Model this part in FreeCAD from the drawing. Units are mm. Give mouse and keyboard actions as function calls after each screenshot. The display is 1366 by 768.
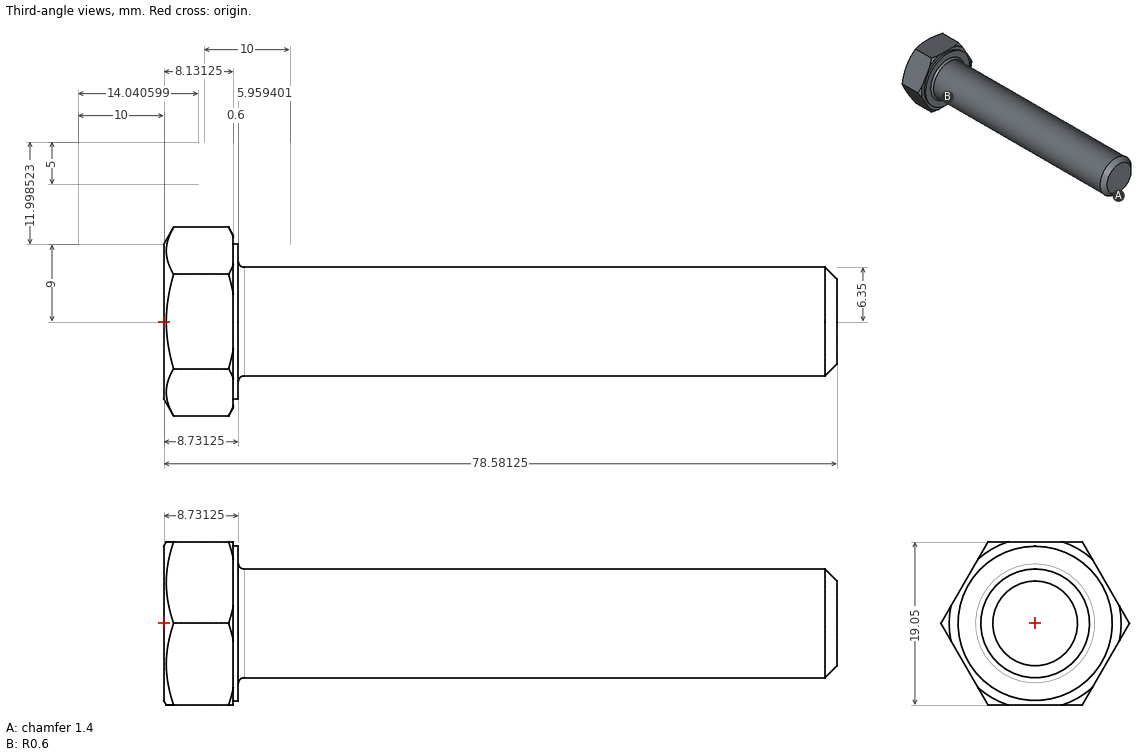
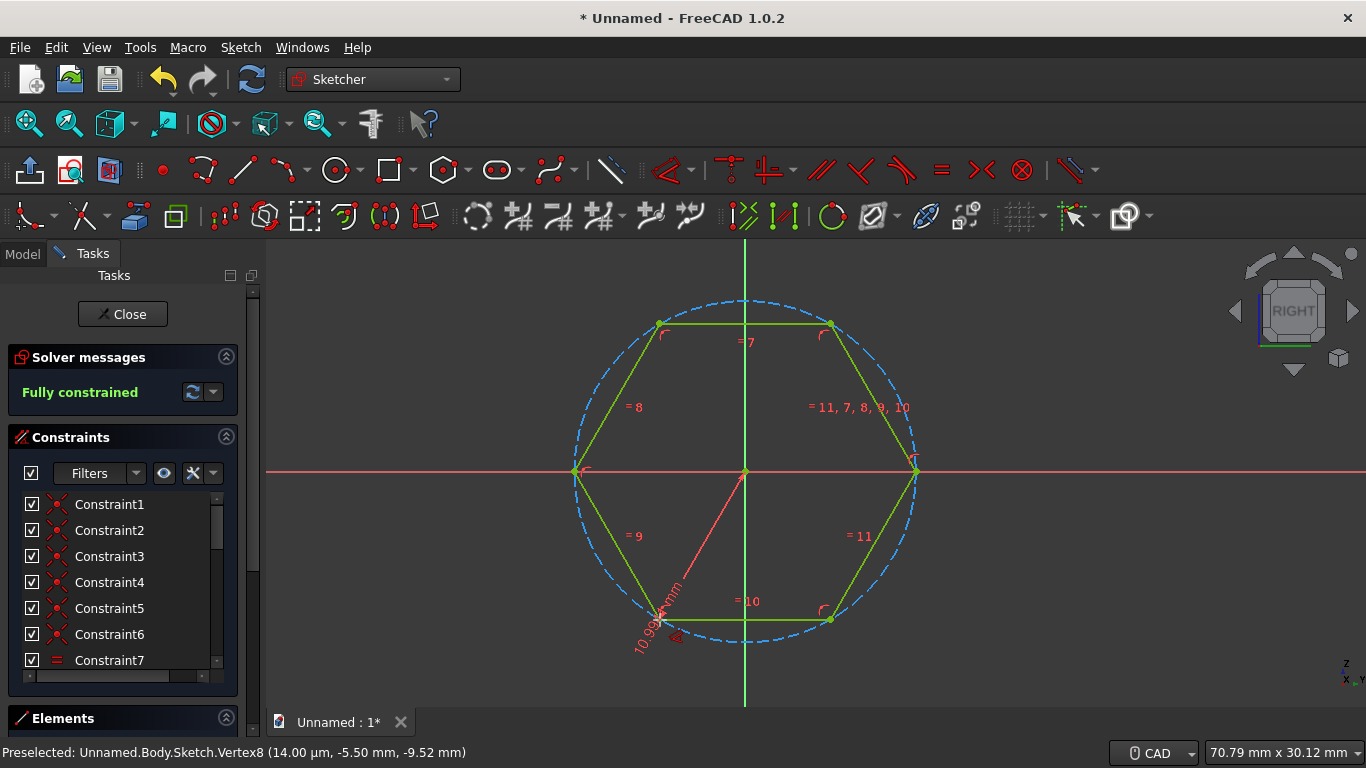
click(831, 324)
click(913, 368)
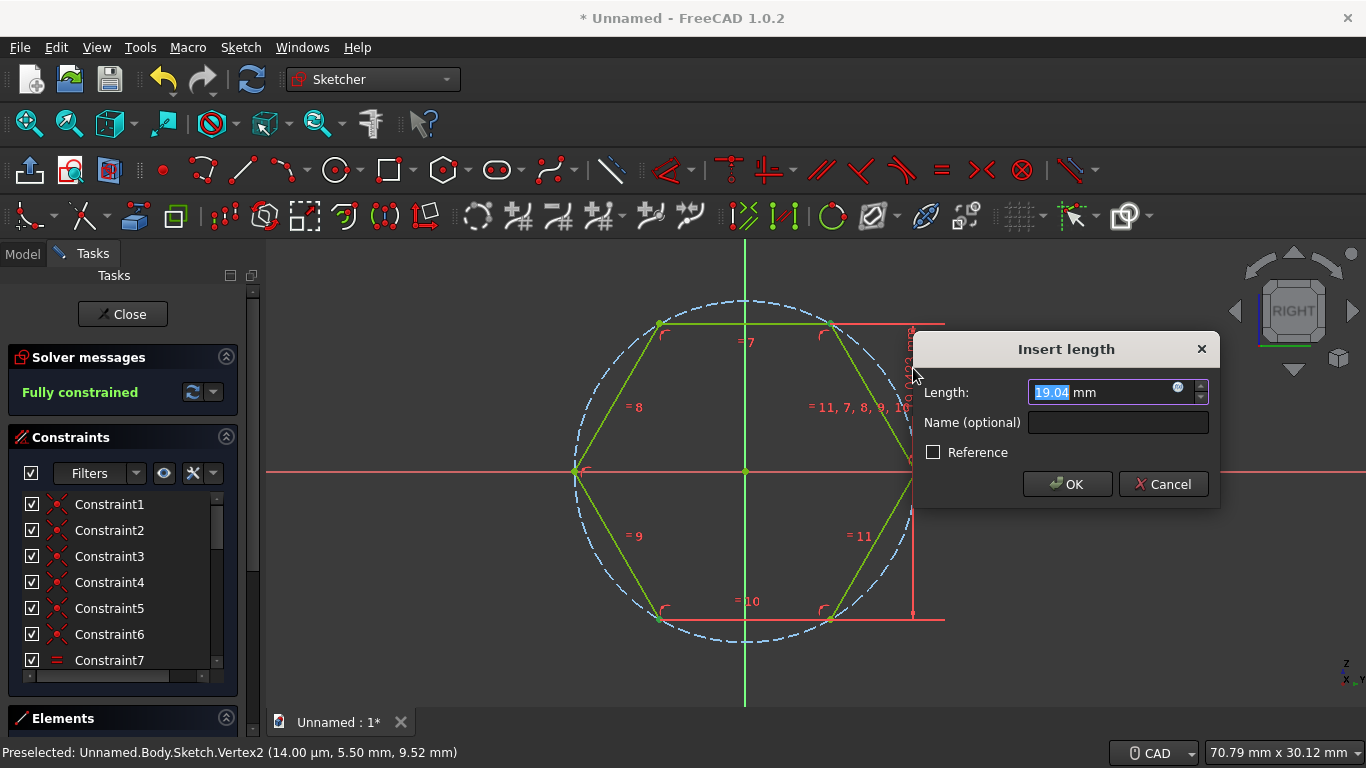
text(19.05)
key(Return)
key(Escape)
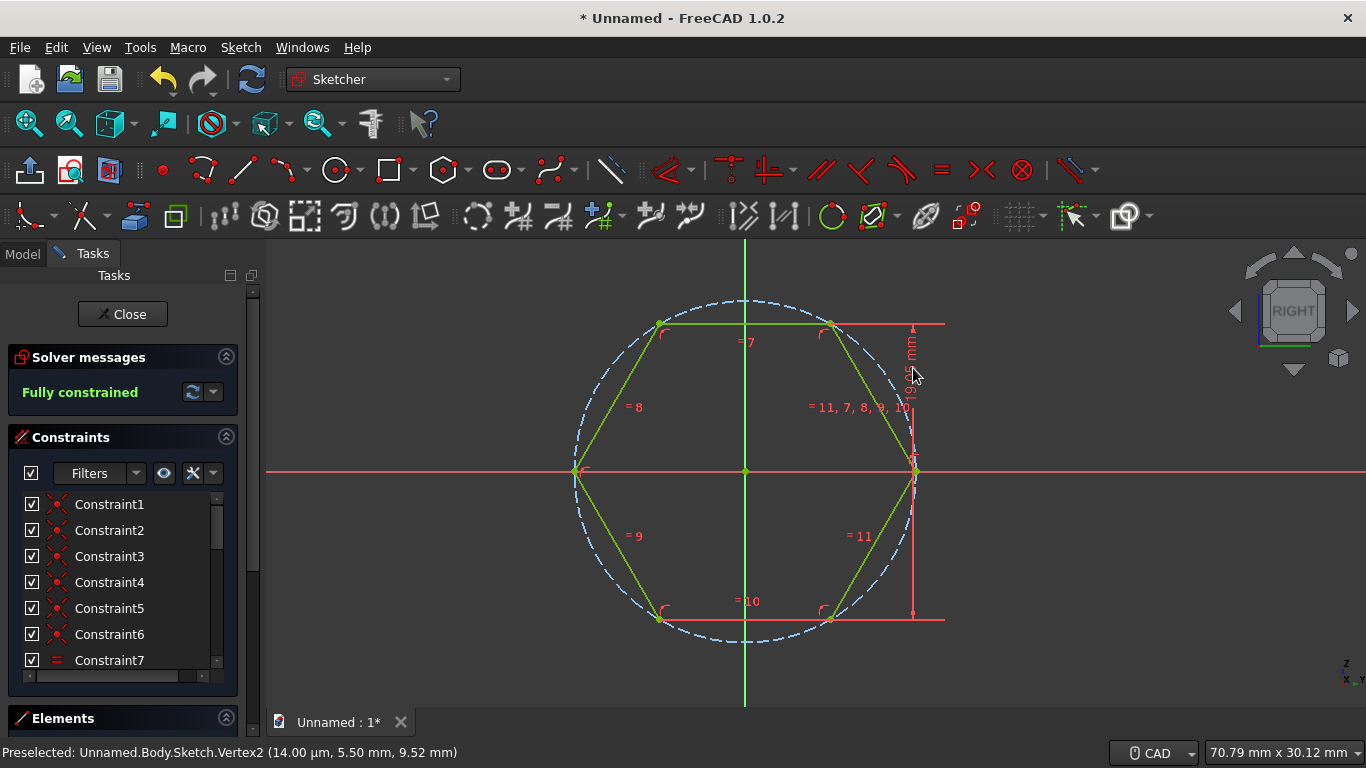
click(123, 314)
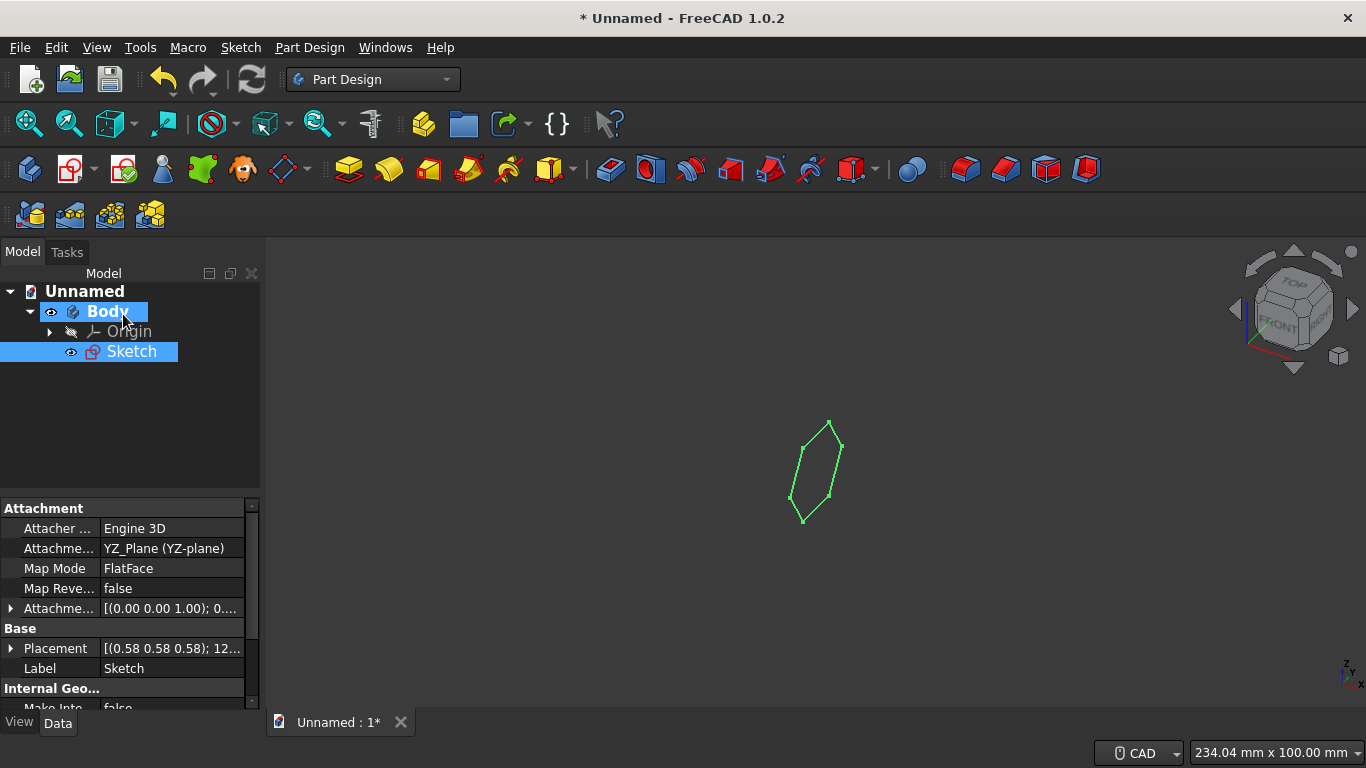
click(350, 170)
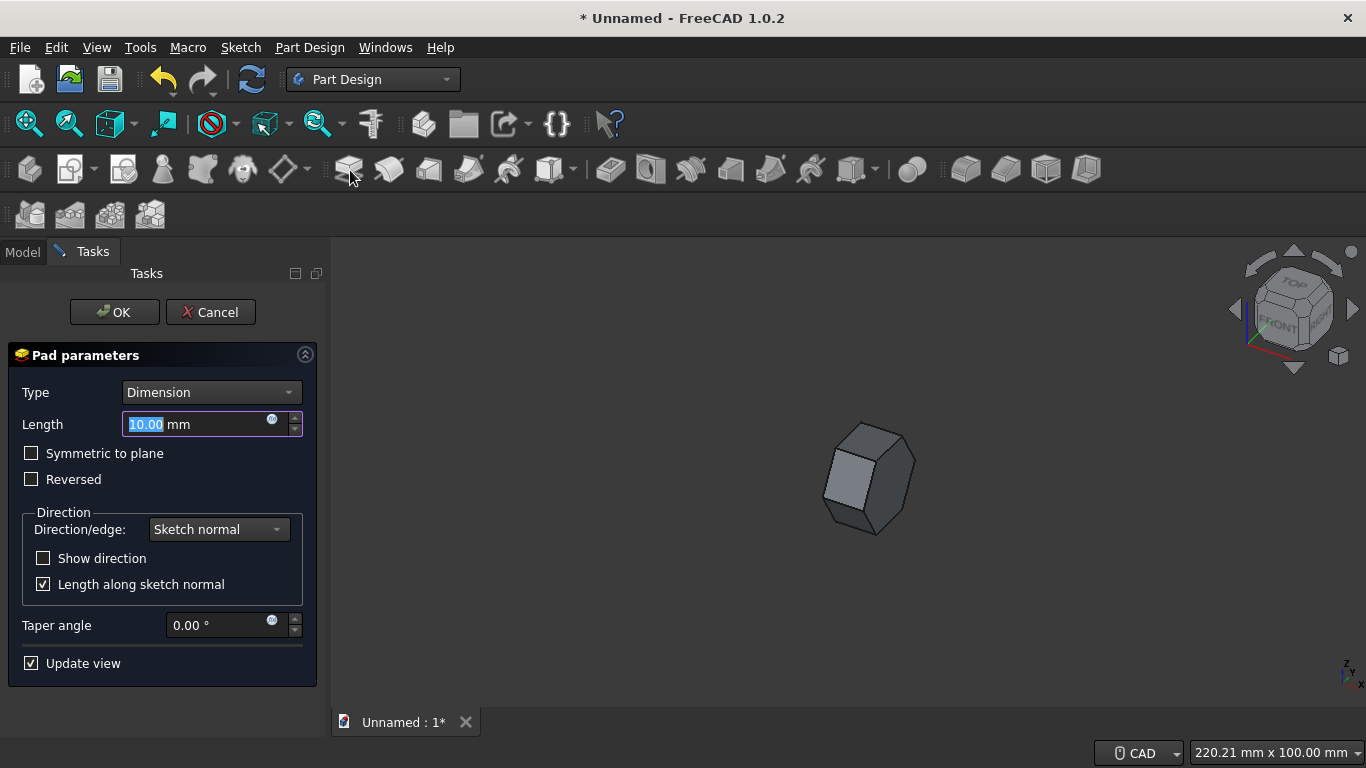
text(8.73125)
key(Tab)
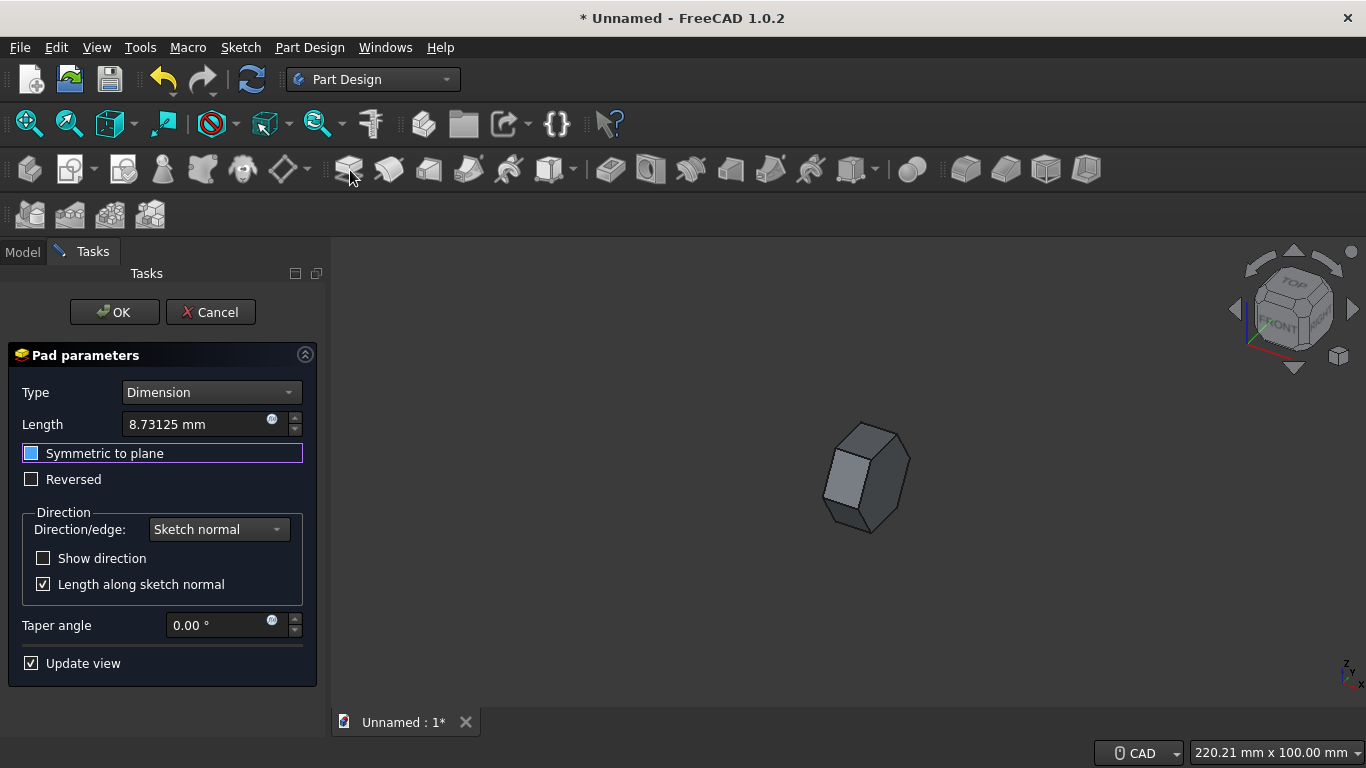
click(115, 312)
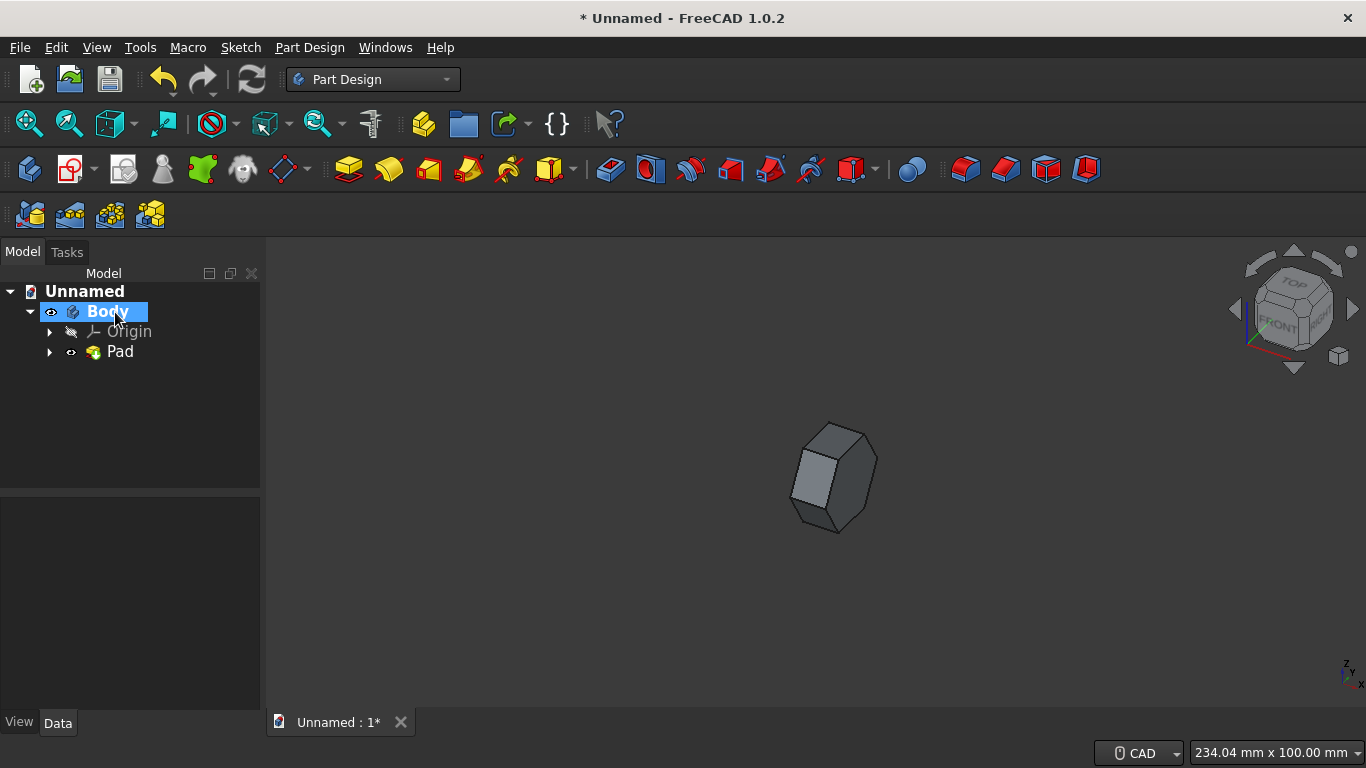
click(30, 124)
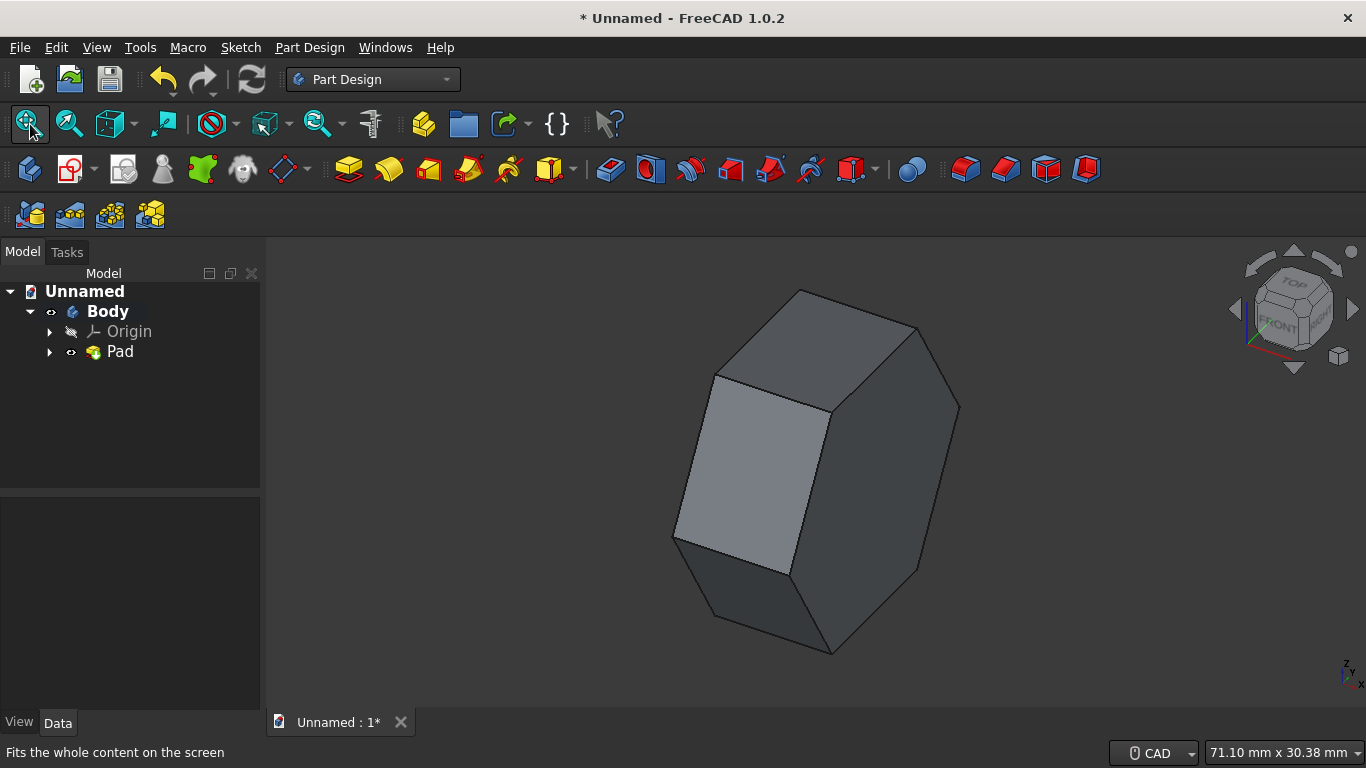
click(70, 170)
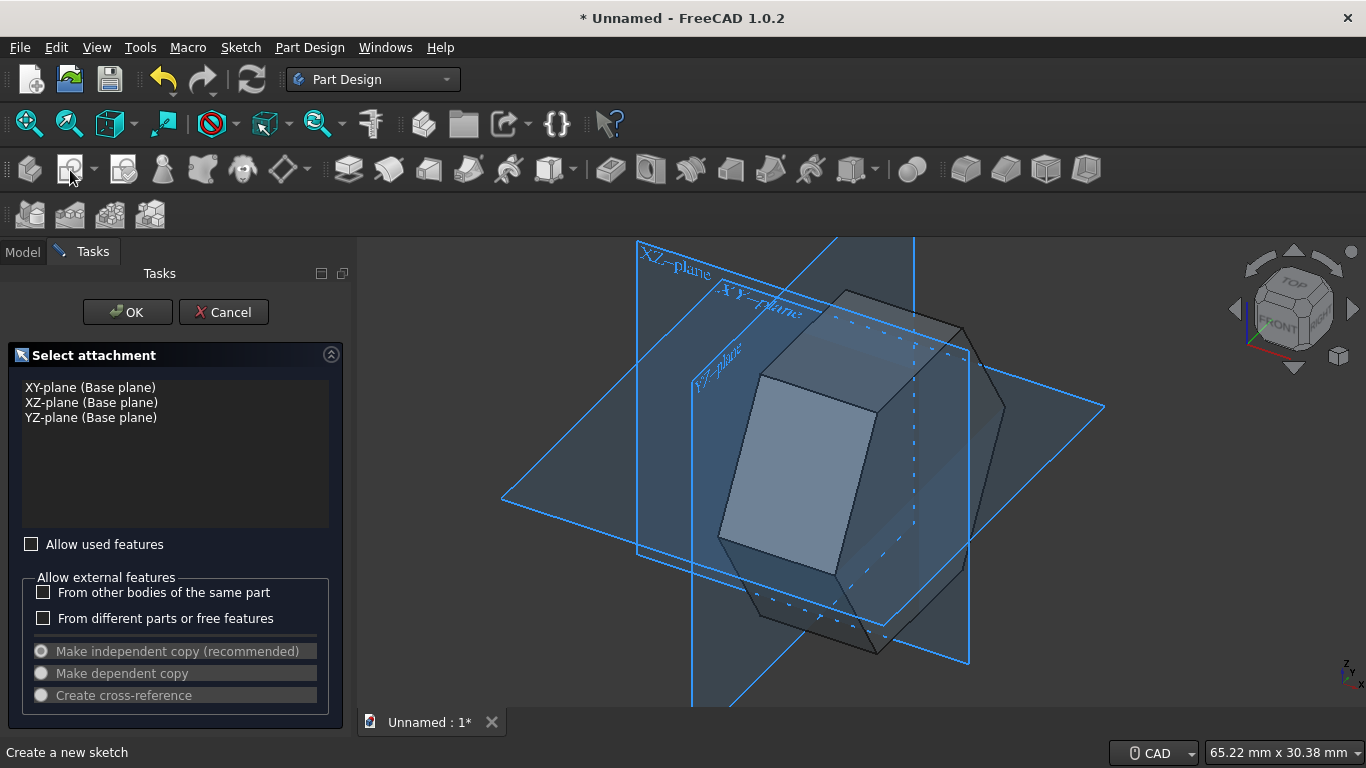
click(82, 388)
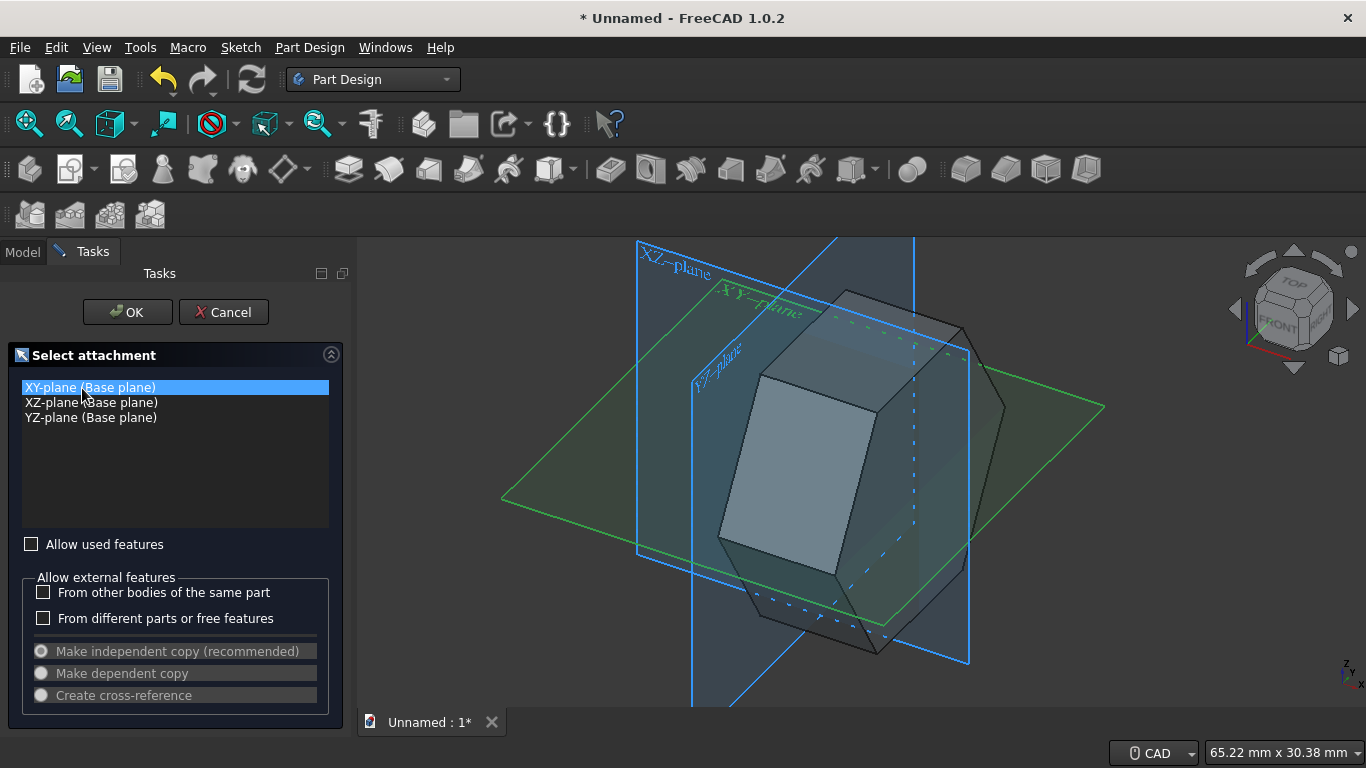
click(128, 312)